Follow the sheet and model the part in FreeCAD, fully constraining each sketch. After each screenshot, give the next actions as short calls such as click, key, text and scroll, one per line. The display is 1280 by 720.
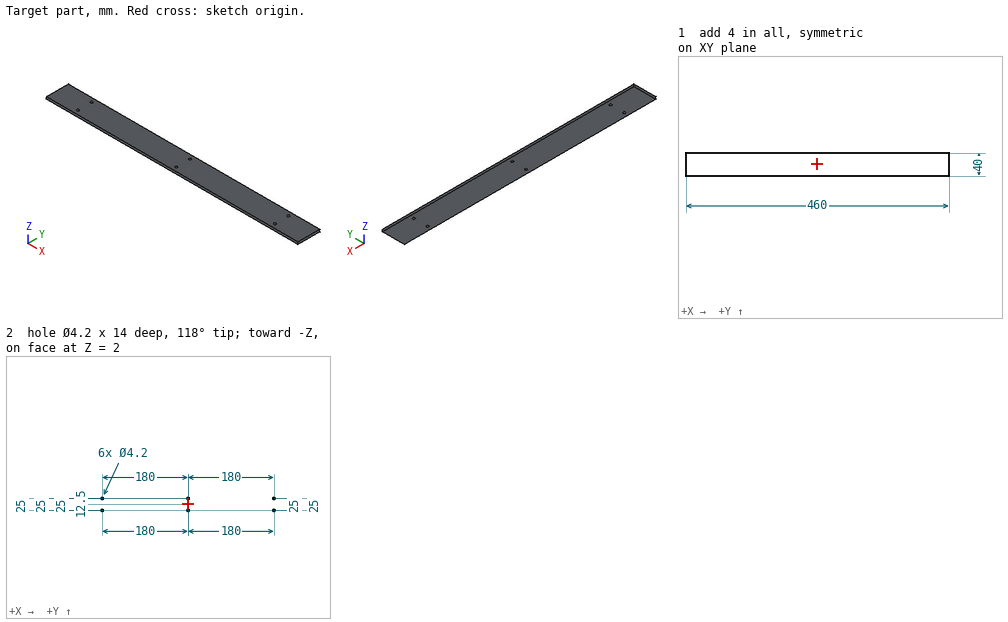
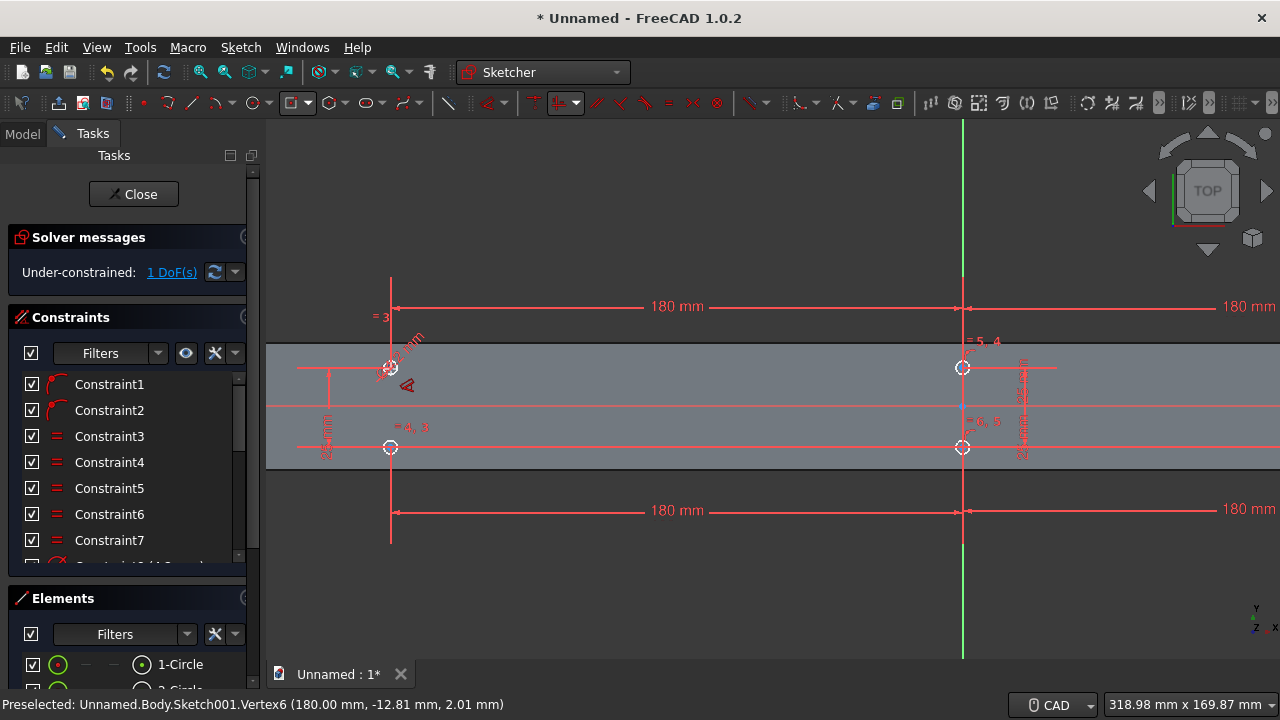
click(391, 368)
click(357, 387)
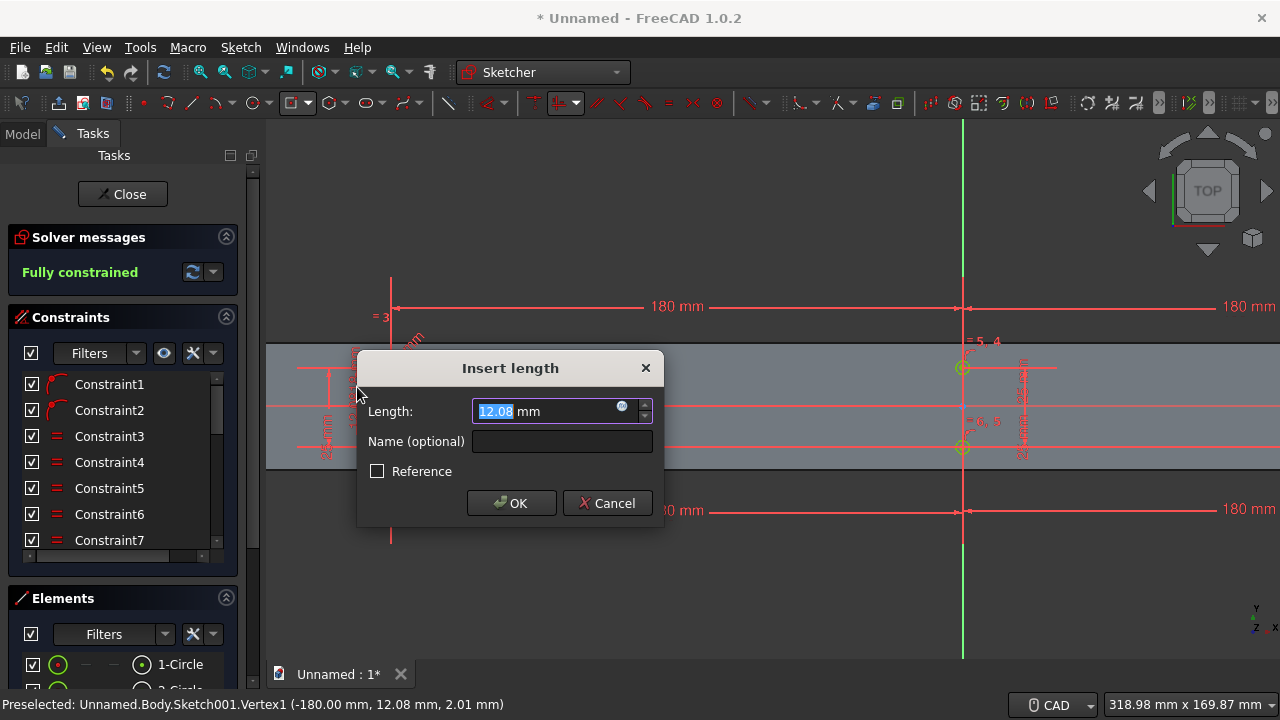
text(12.5)
key(Return)
key(Escape)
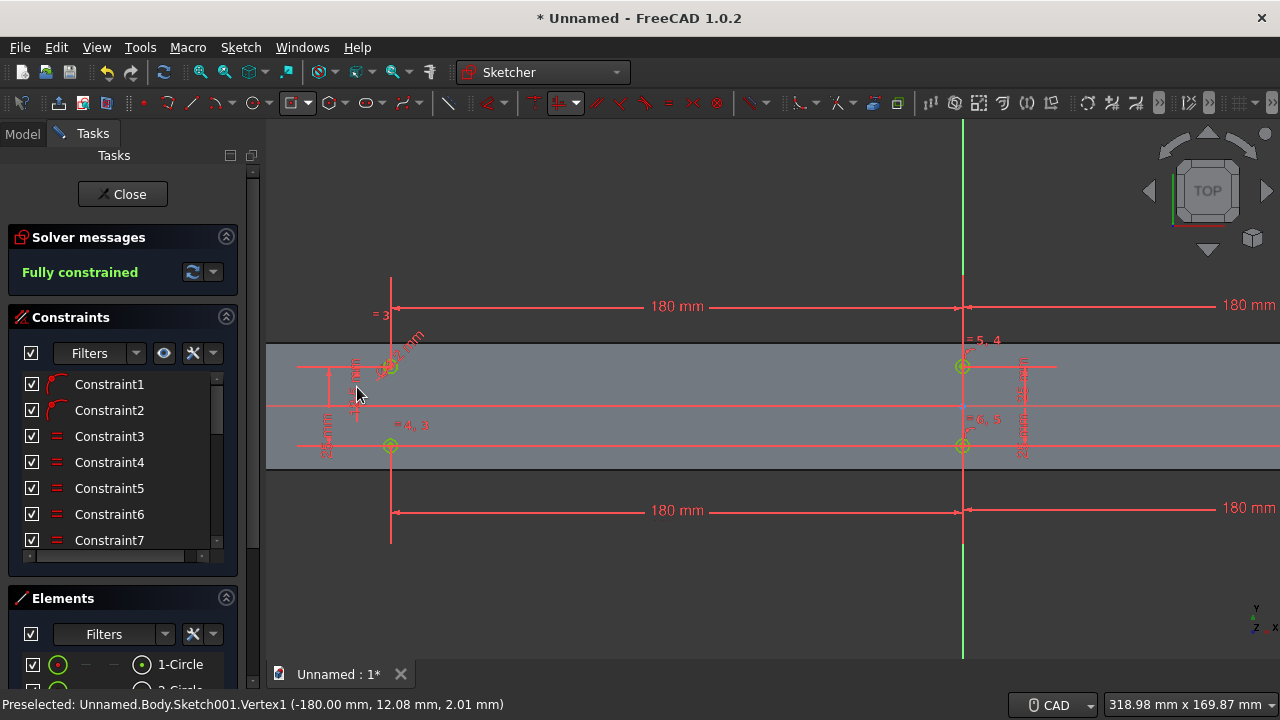
click(123, 194)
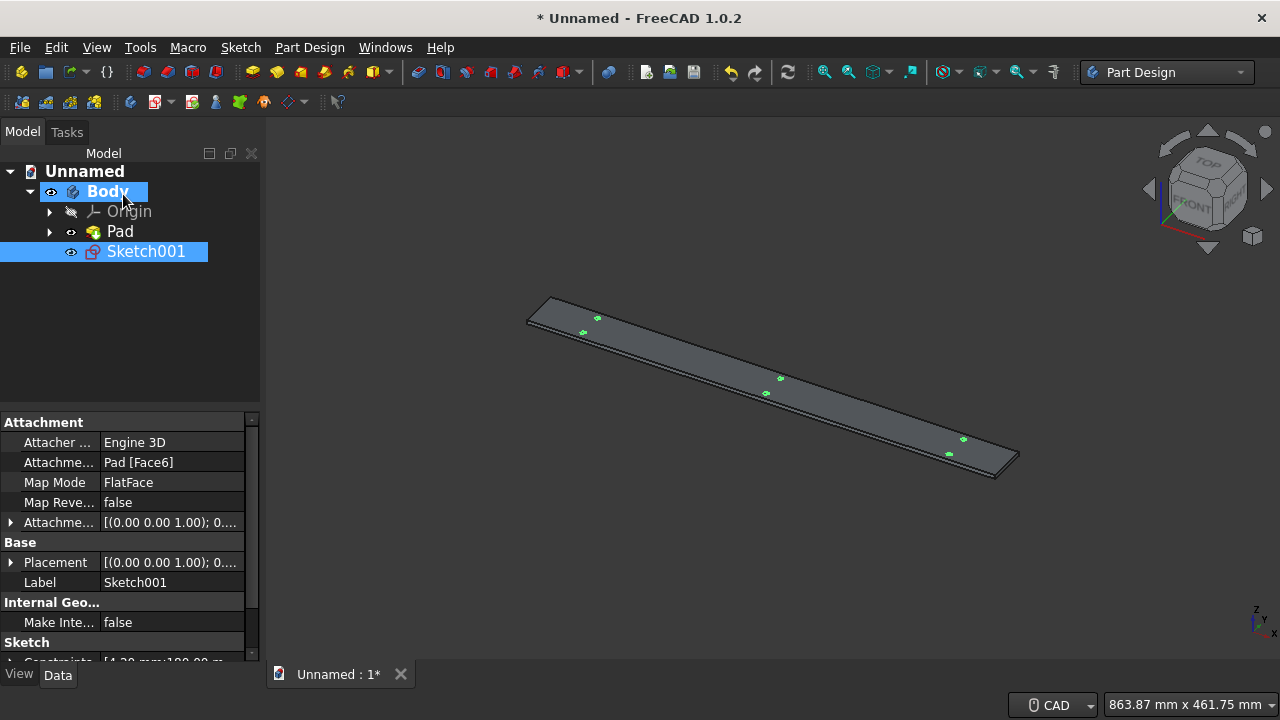
click(444, 72)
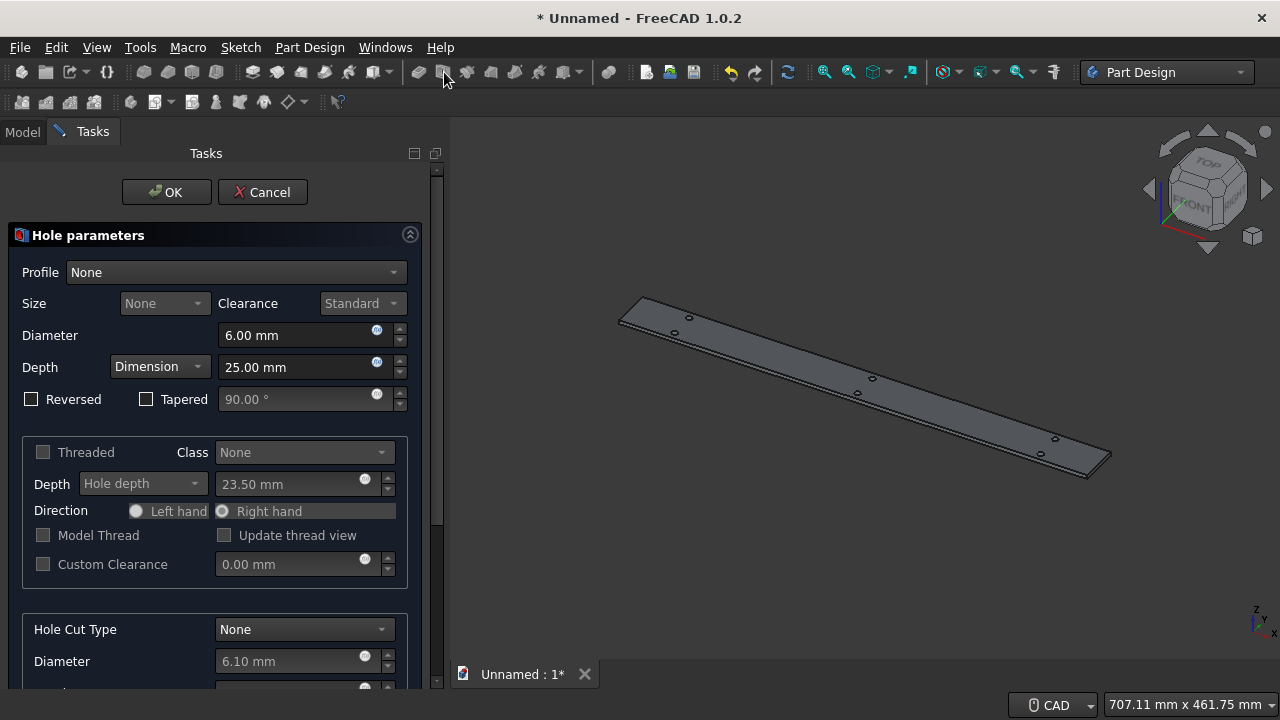
triple_click(305, 335)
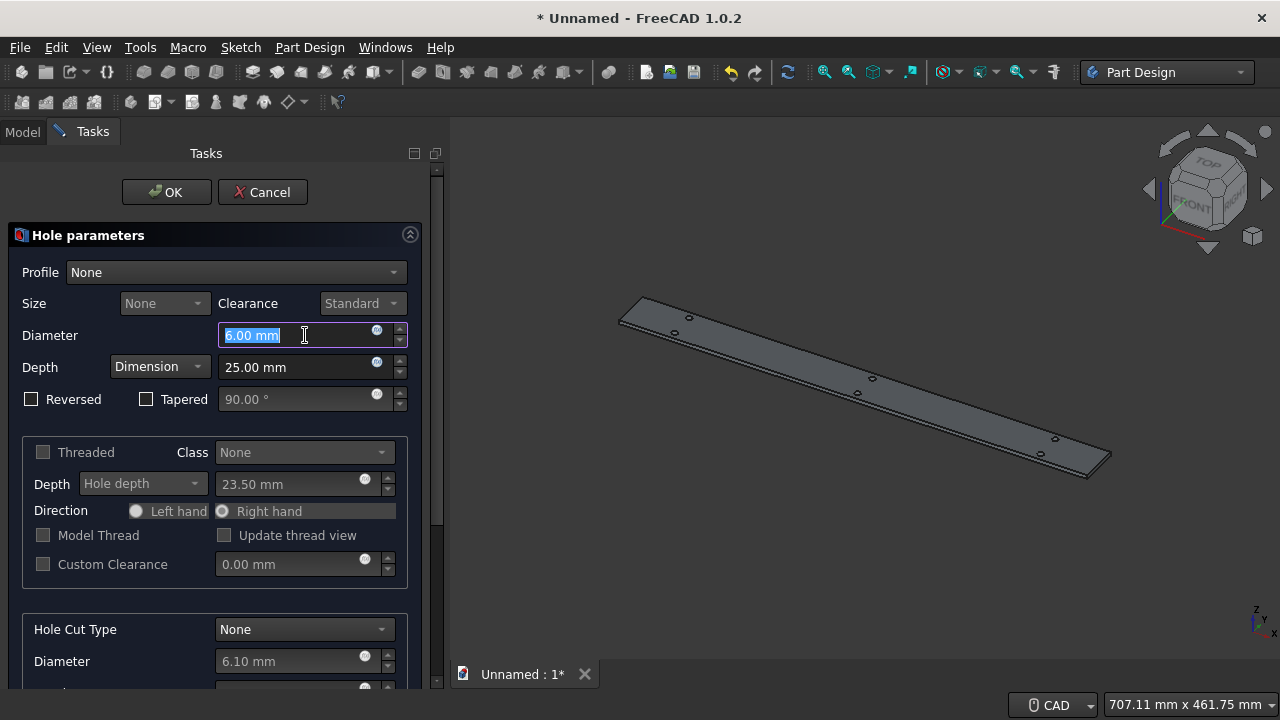
text(4.2)
key(Tab)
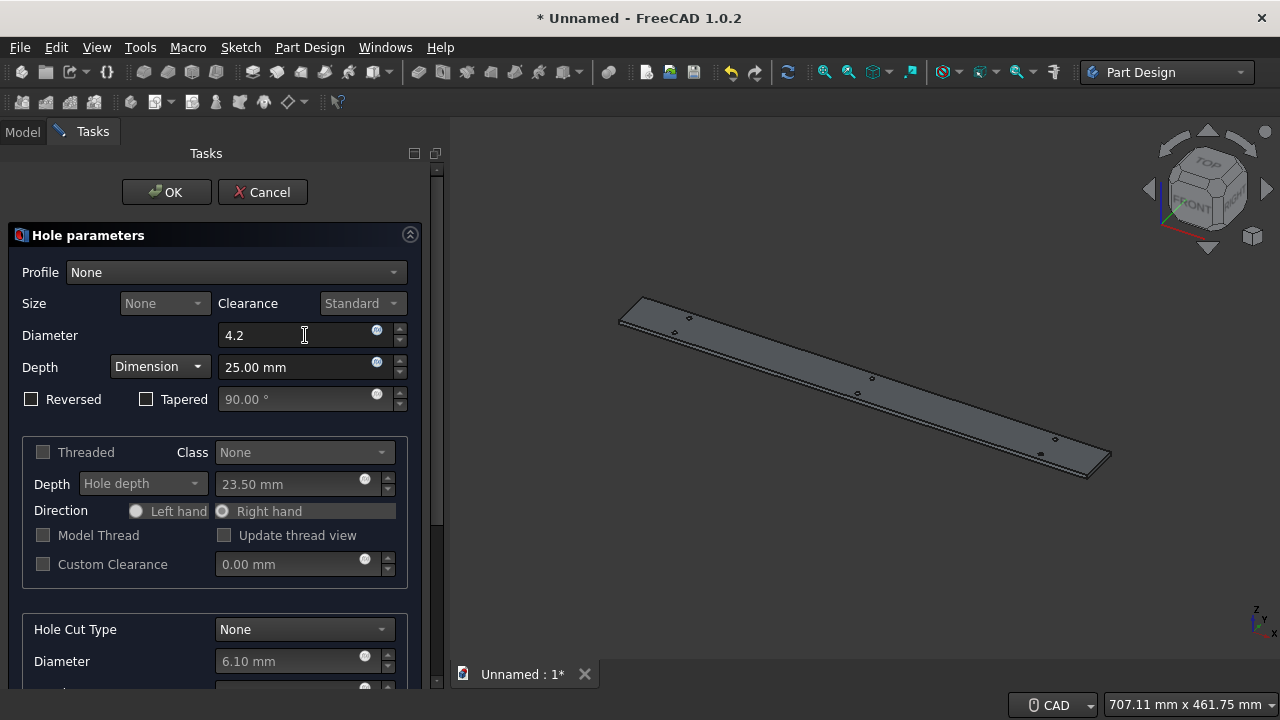
triple_click(305, 367)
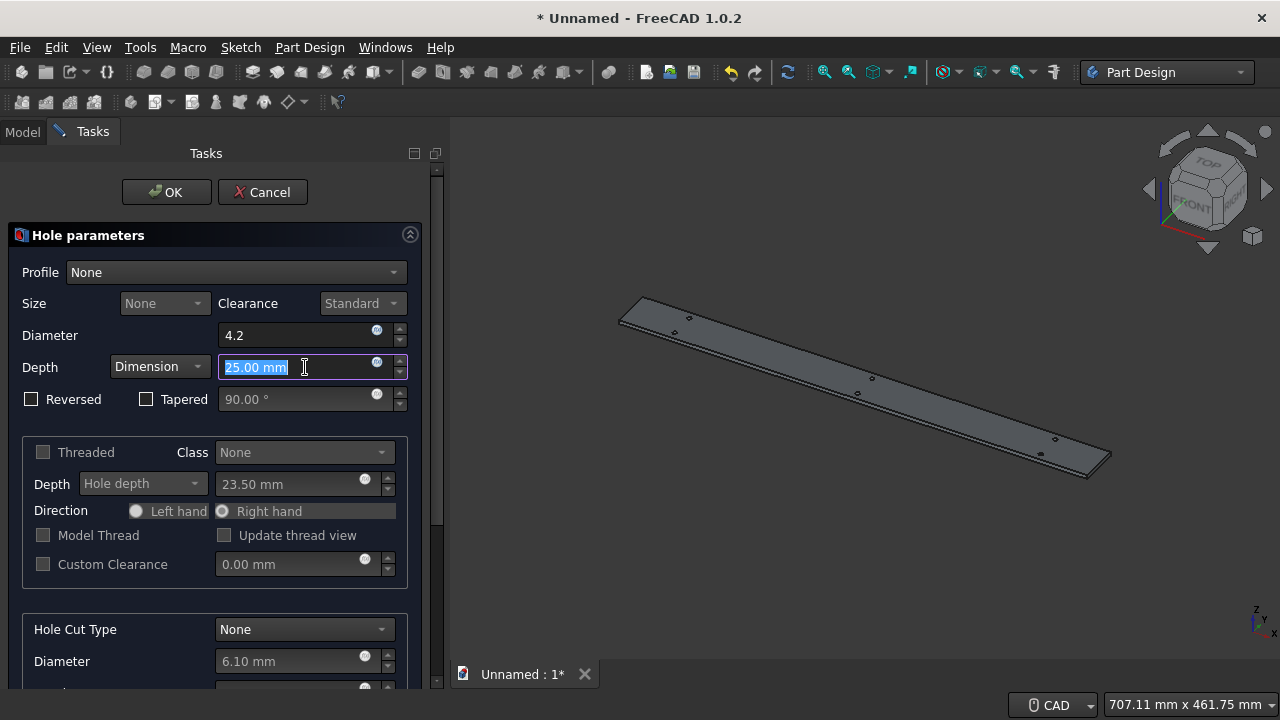
text(14)
key(Tab)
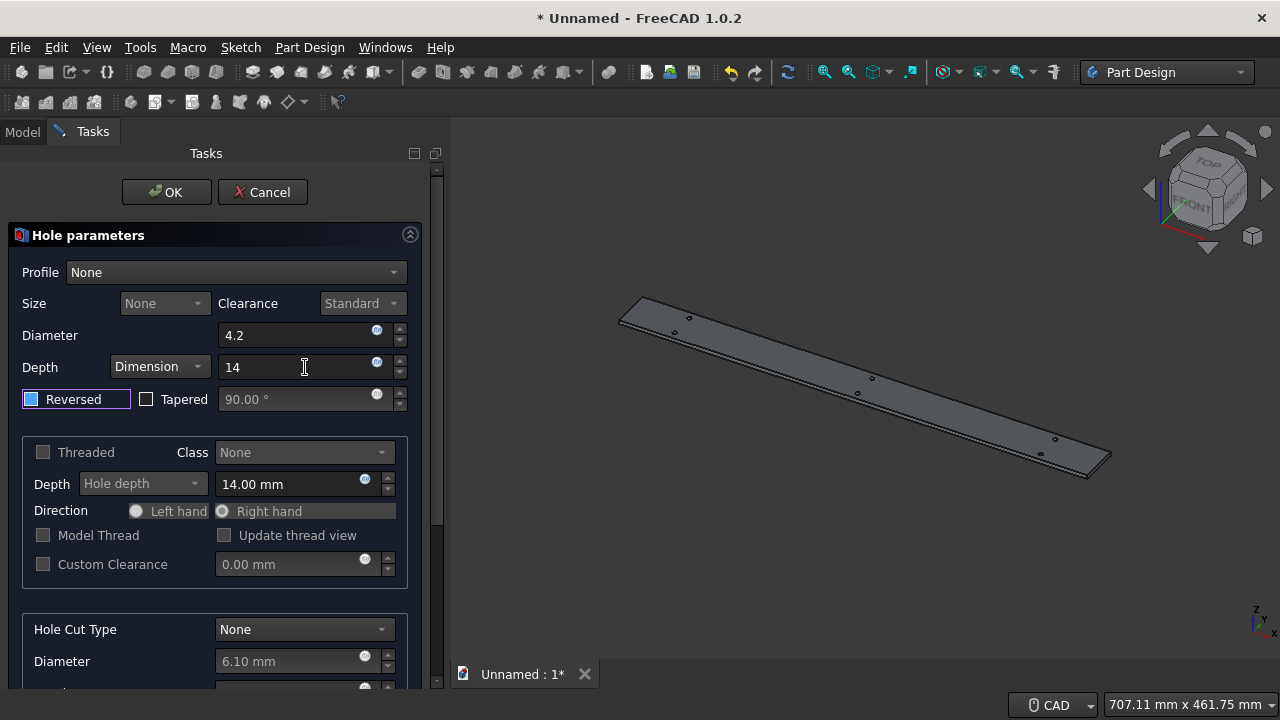
click(167, 192)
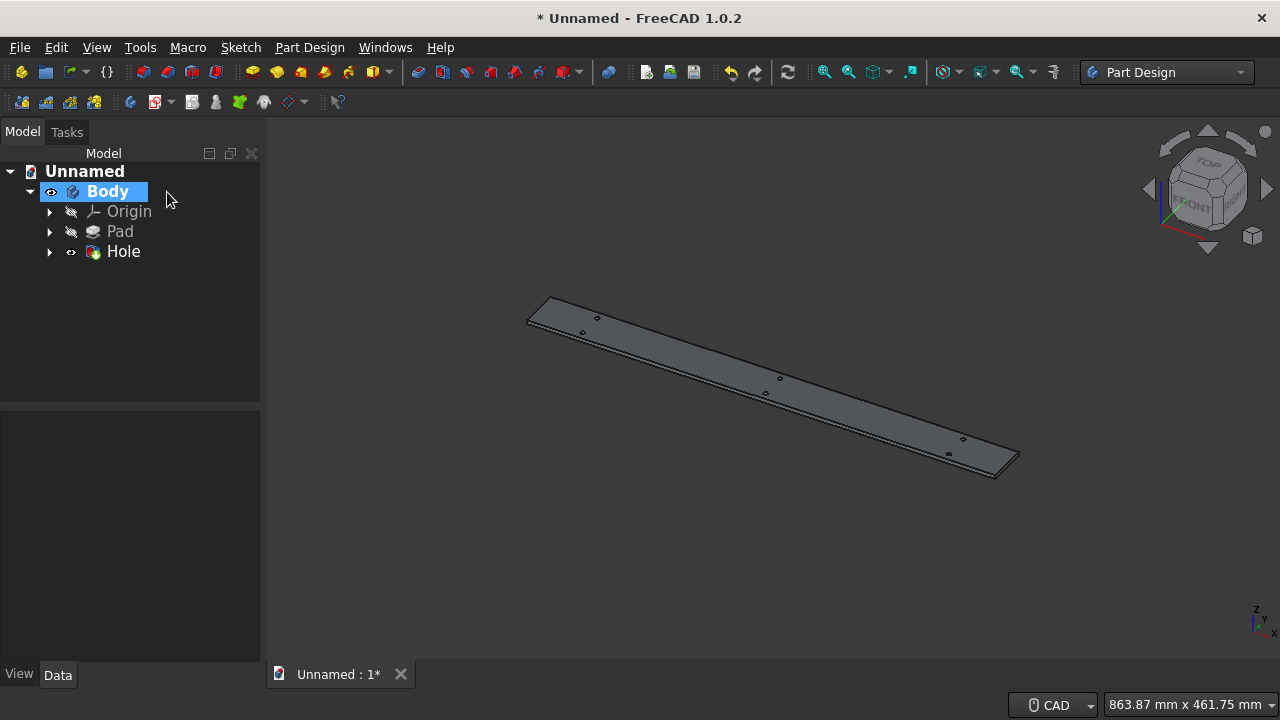
key(0)